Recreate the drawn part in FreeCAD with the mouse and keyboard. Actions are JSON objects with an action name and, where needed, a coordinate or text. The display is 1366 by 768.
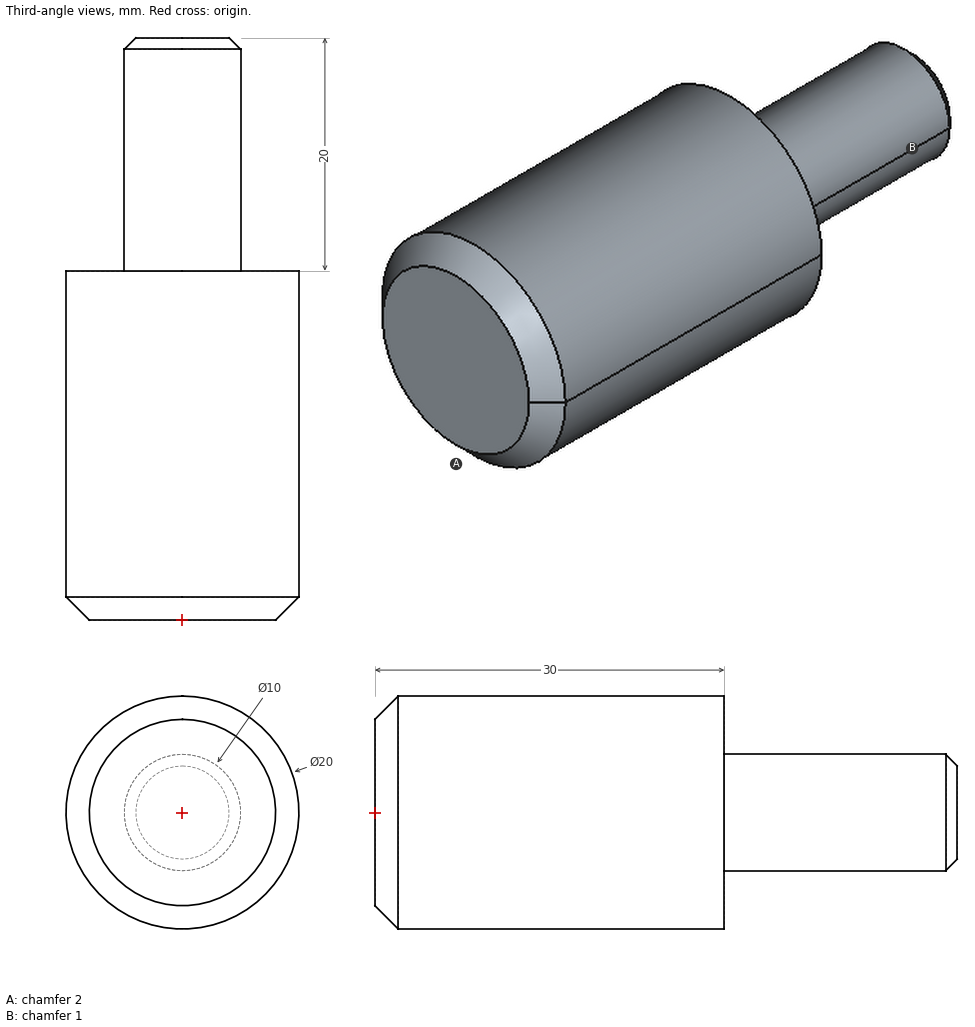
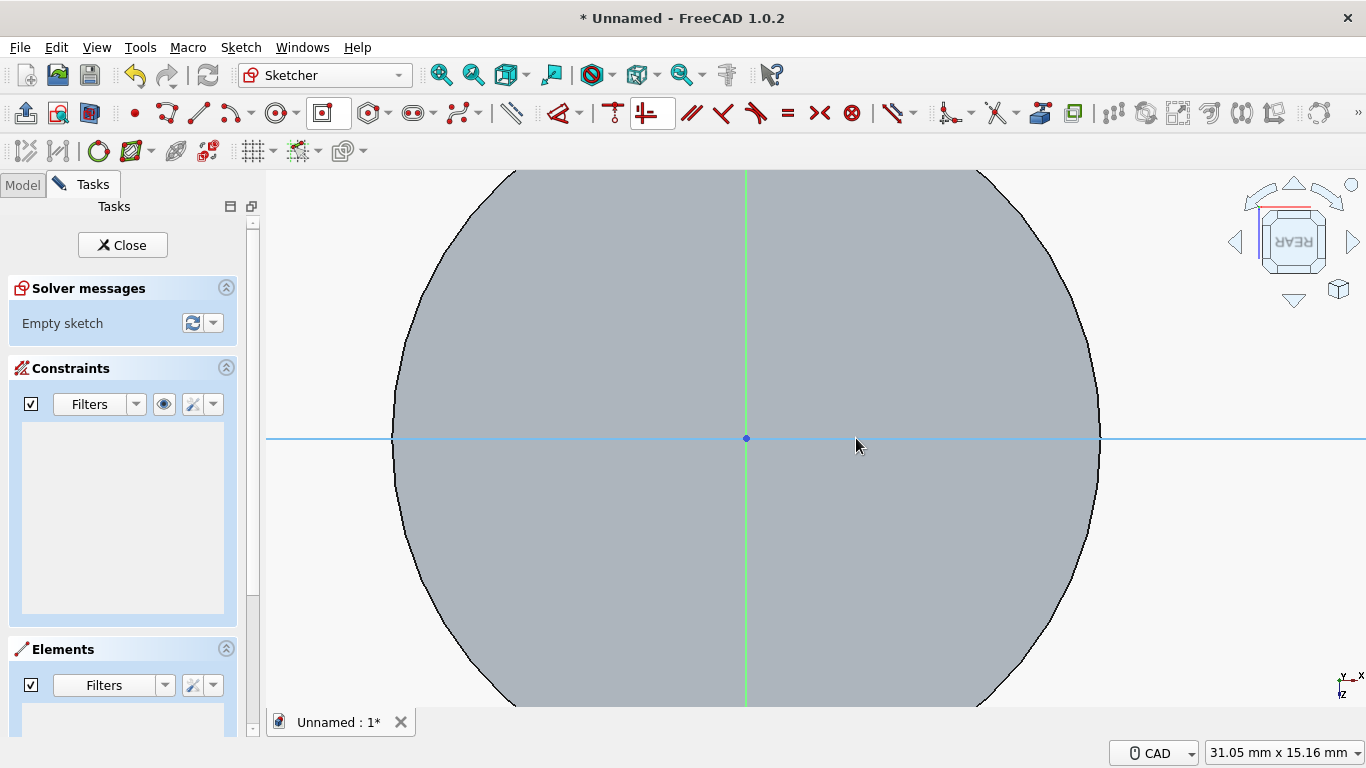
{"action": "left_click", "coordinate": [276, 114]}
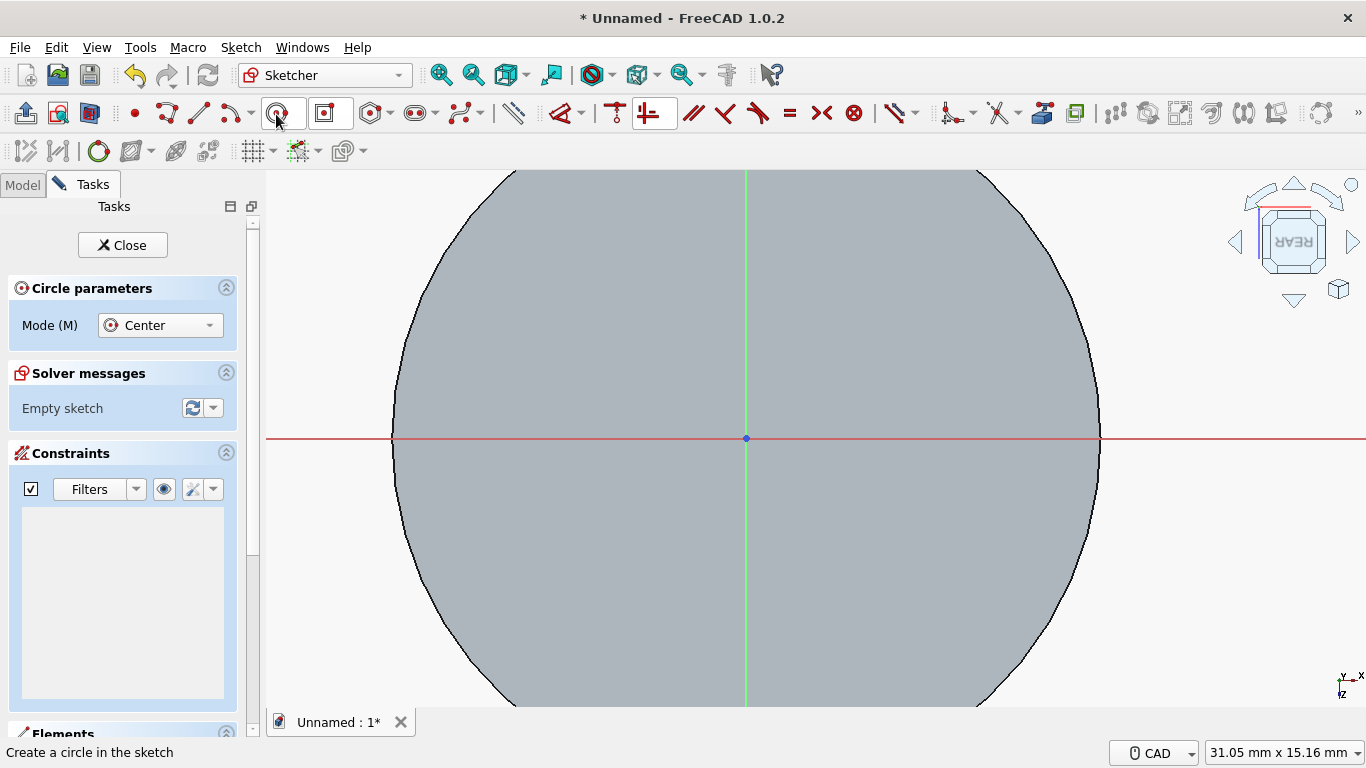
{"action": "left_click", "coordinate": [746, 438]}
{"action": "mouse_move", "coordinate": [872, 313]}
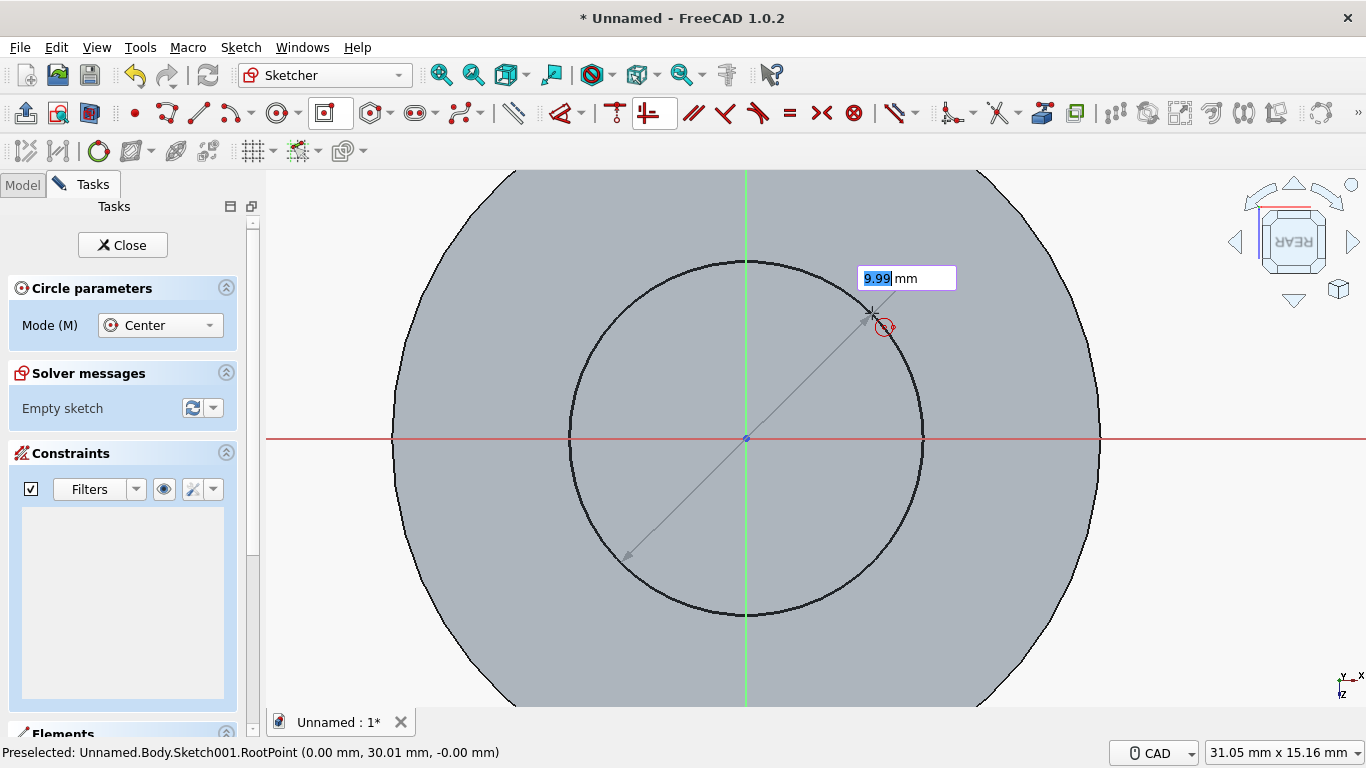
{"action": "type", "text": "10"}
{"action": "key", "text": "Return"}
{"action": "key", "text": "Escape"}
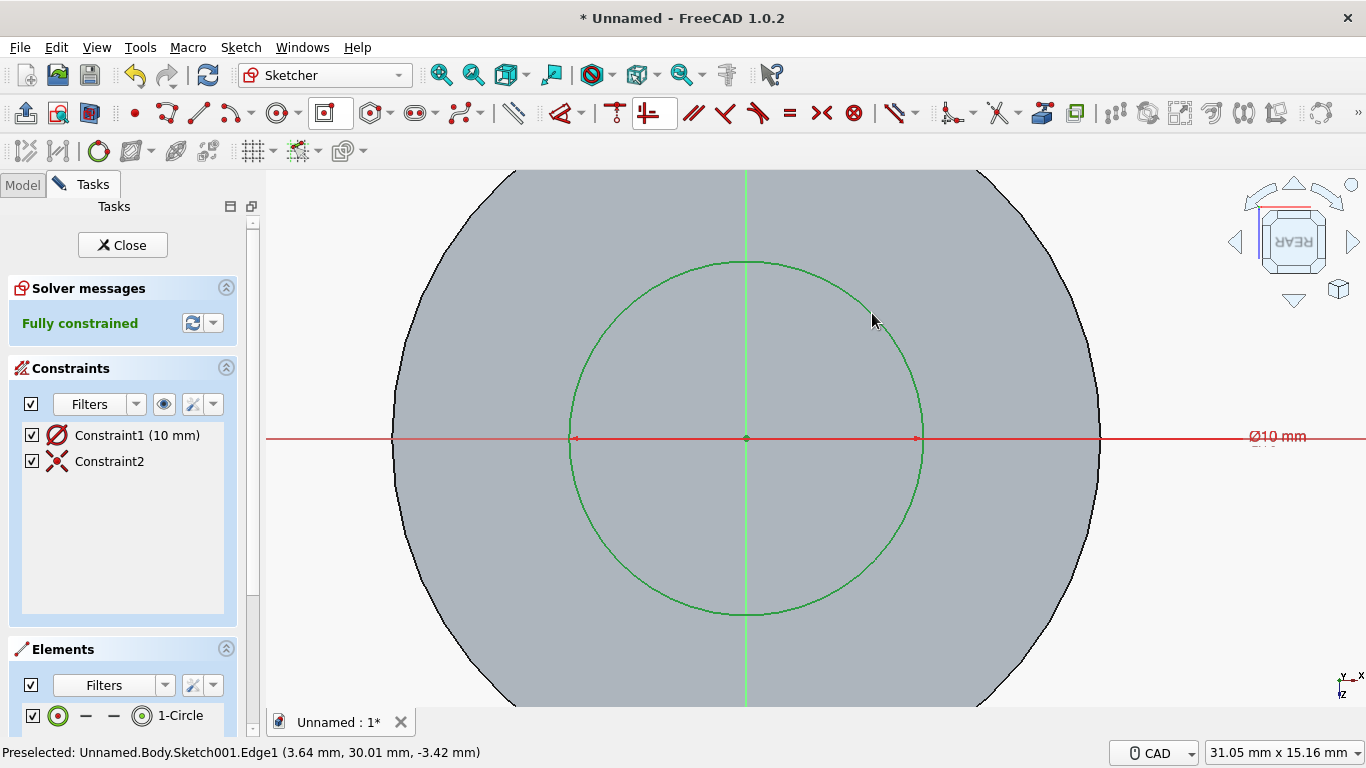
{"action": "left_click", "coordinate": [123, 245]}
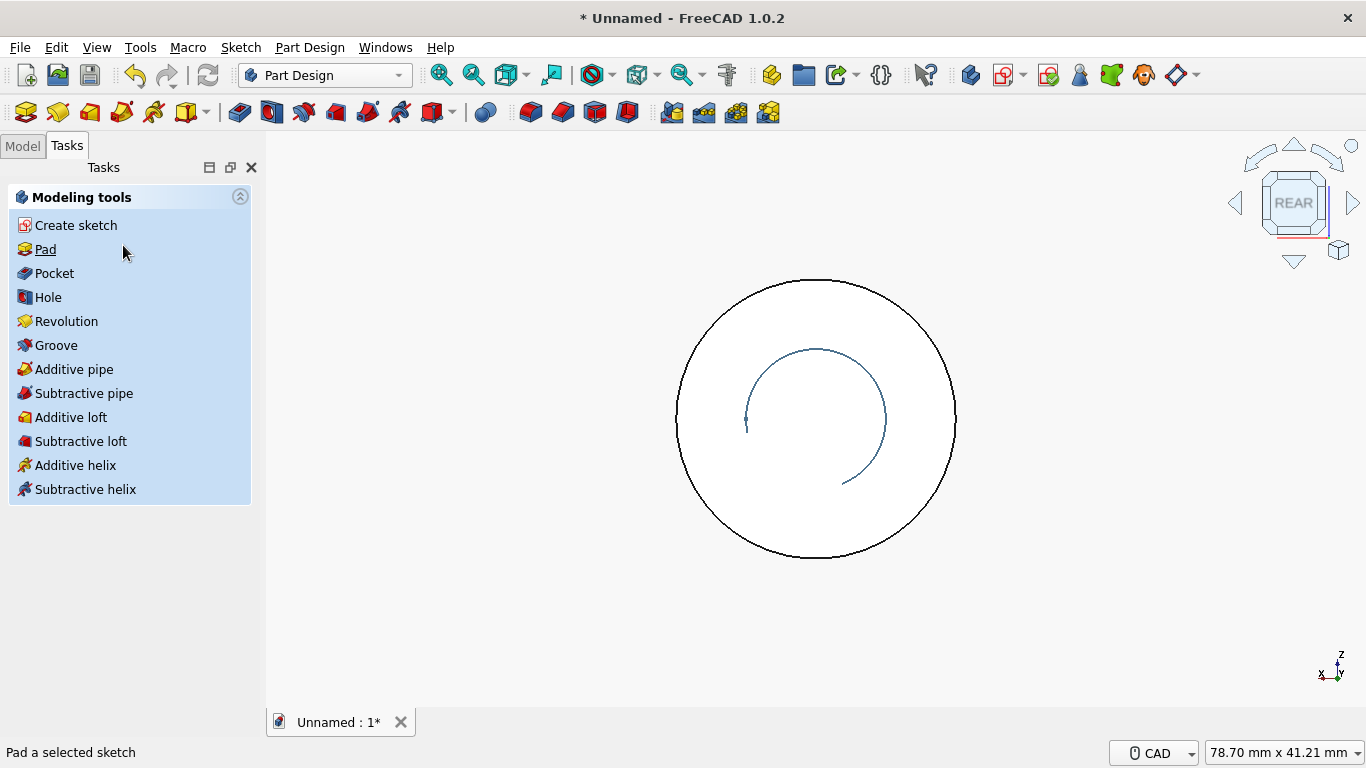
{"action": "left_click", "coordinate": [26, 112]}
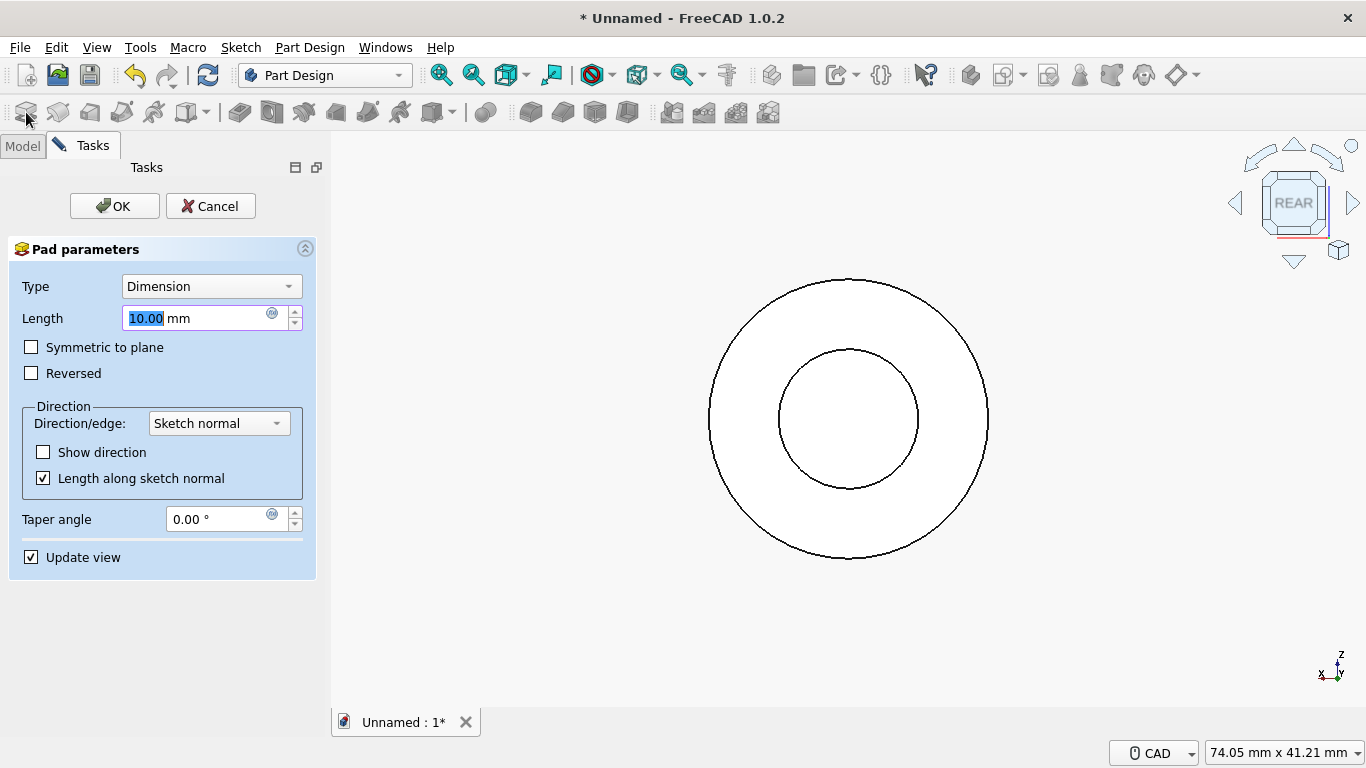
{"action": "type", "text": "20"}
{"action": "key", "text": "Tab"}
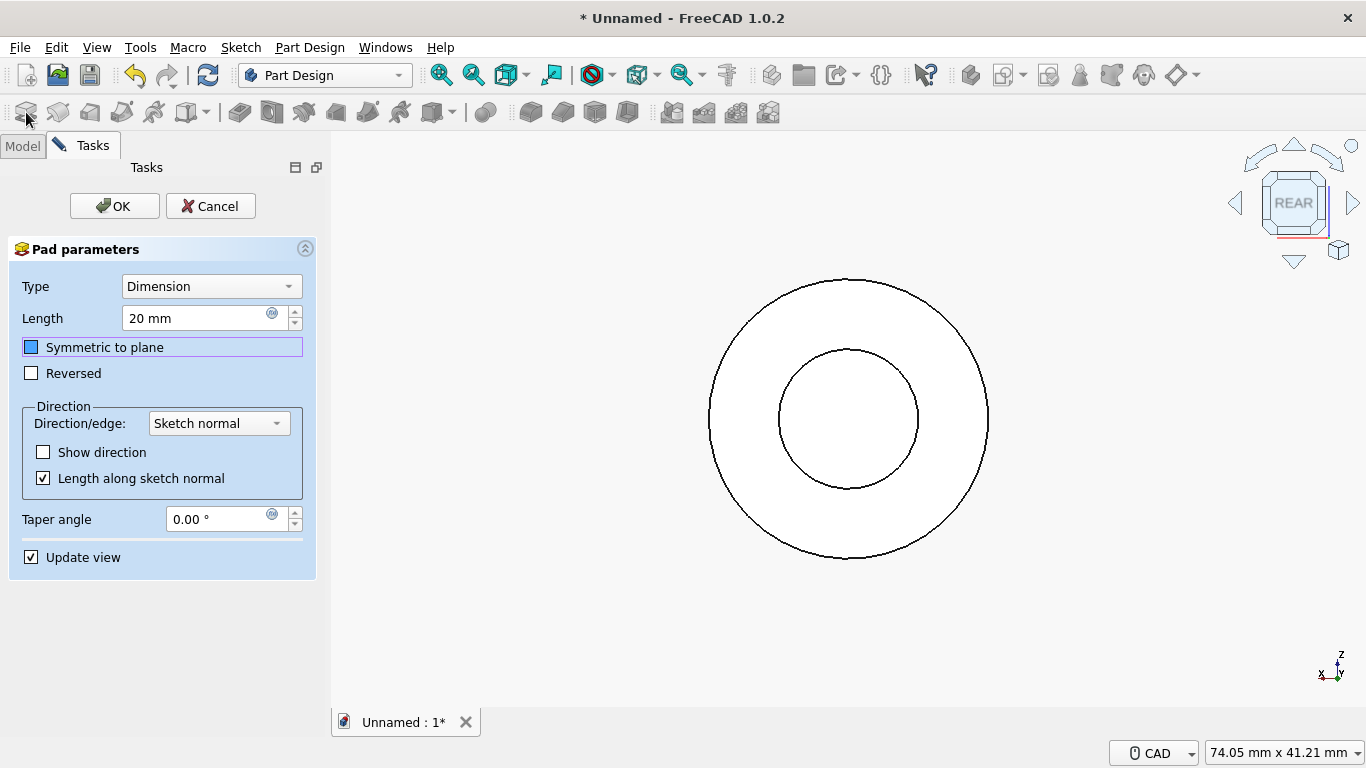
{"action": "left_click", "coordinate": [115, 206]}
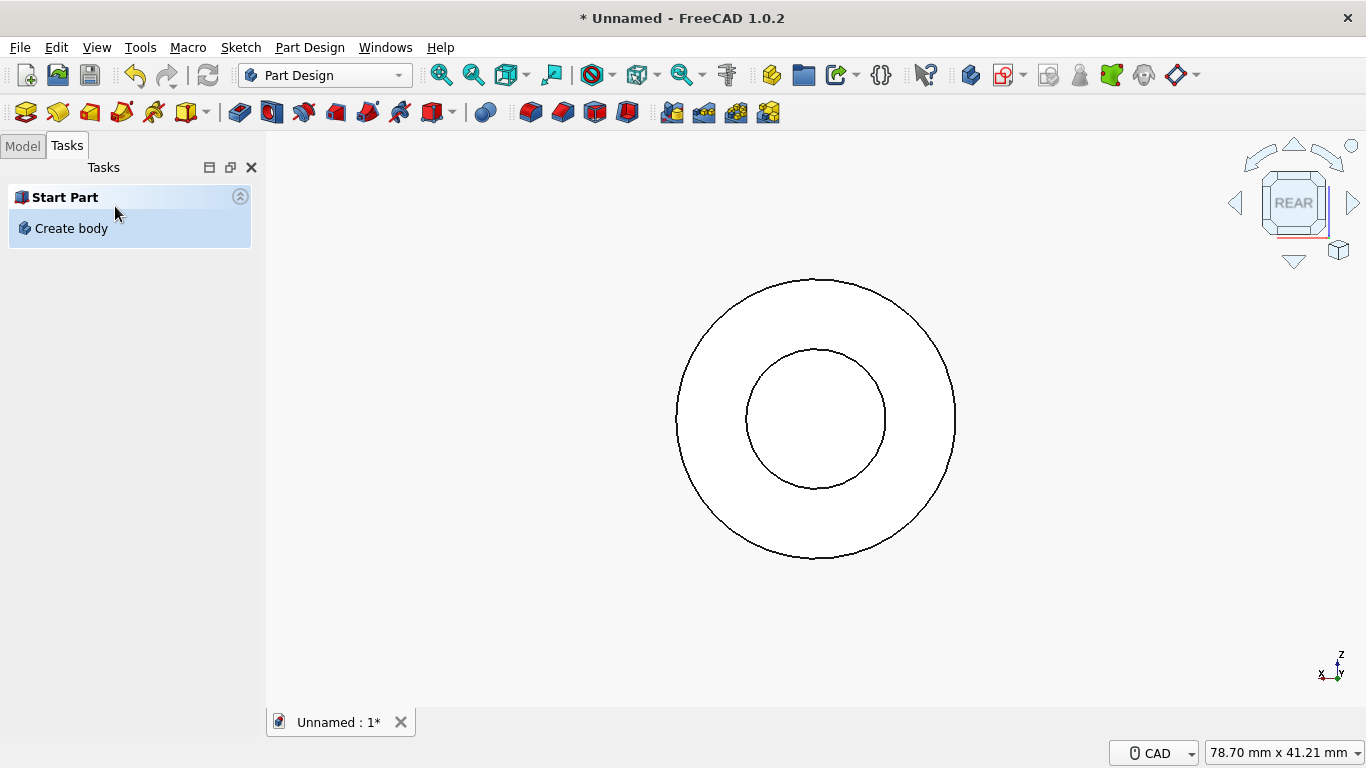
{"action": "key", "text": "0"}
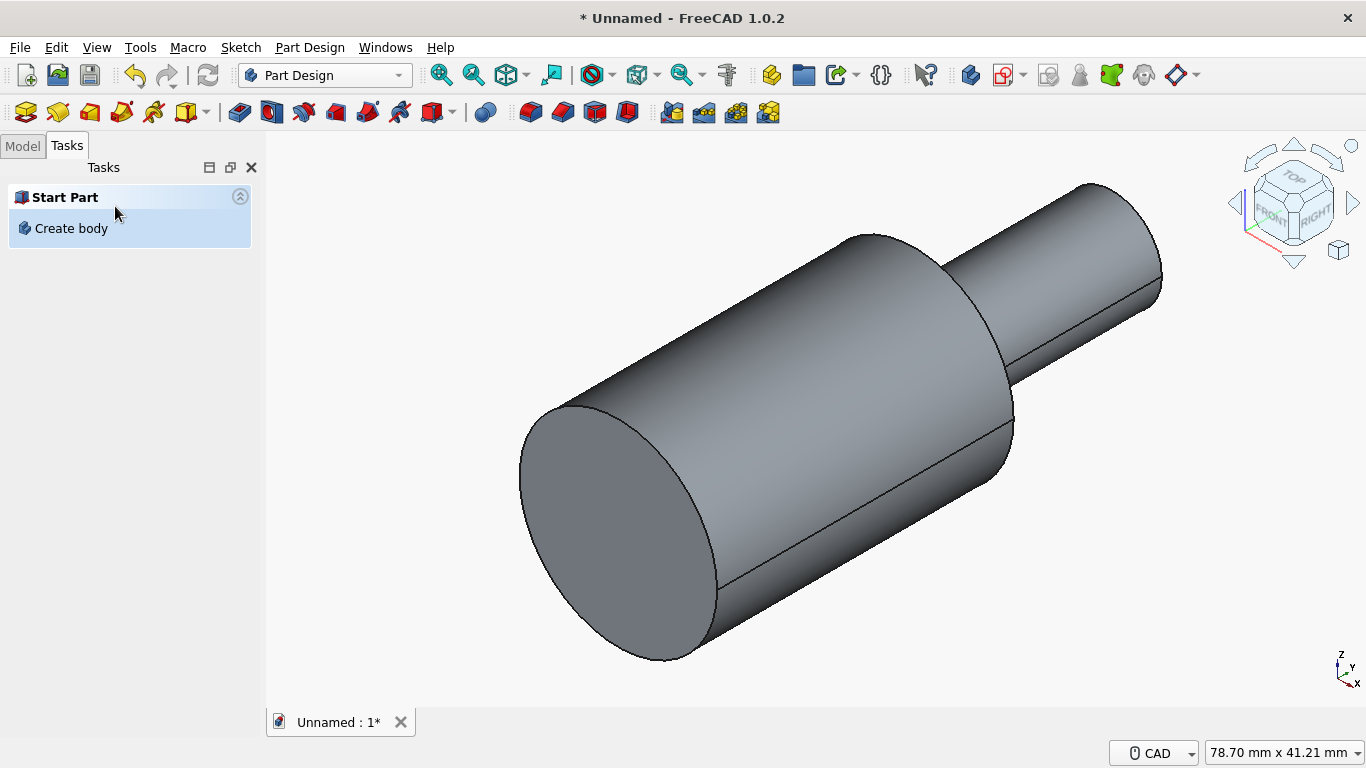
{"action": "left_click", "coordinate": [442, 76]}